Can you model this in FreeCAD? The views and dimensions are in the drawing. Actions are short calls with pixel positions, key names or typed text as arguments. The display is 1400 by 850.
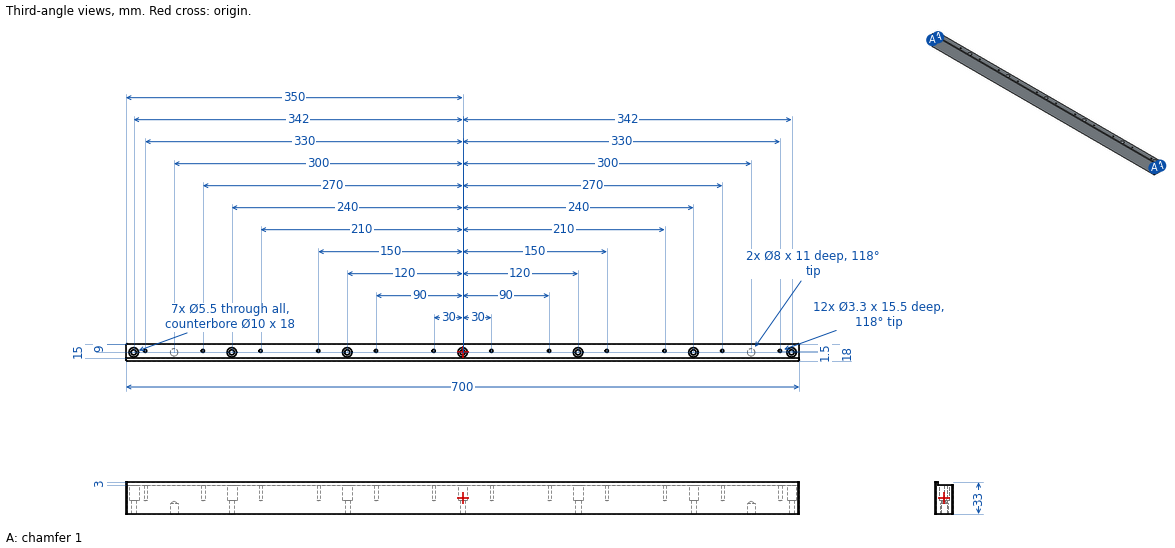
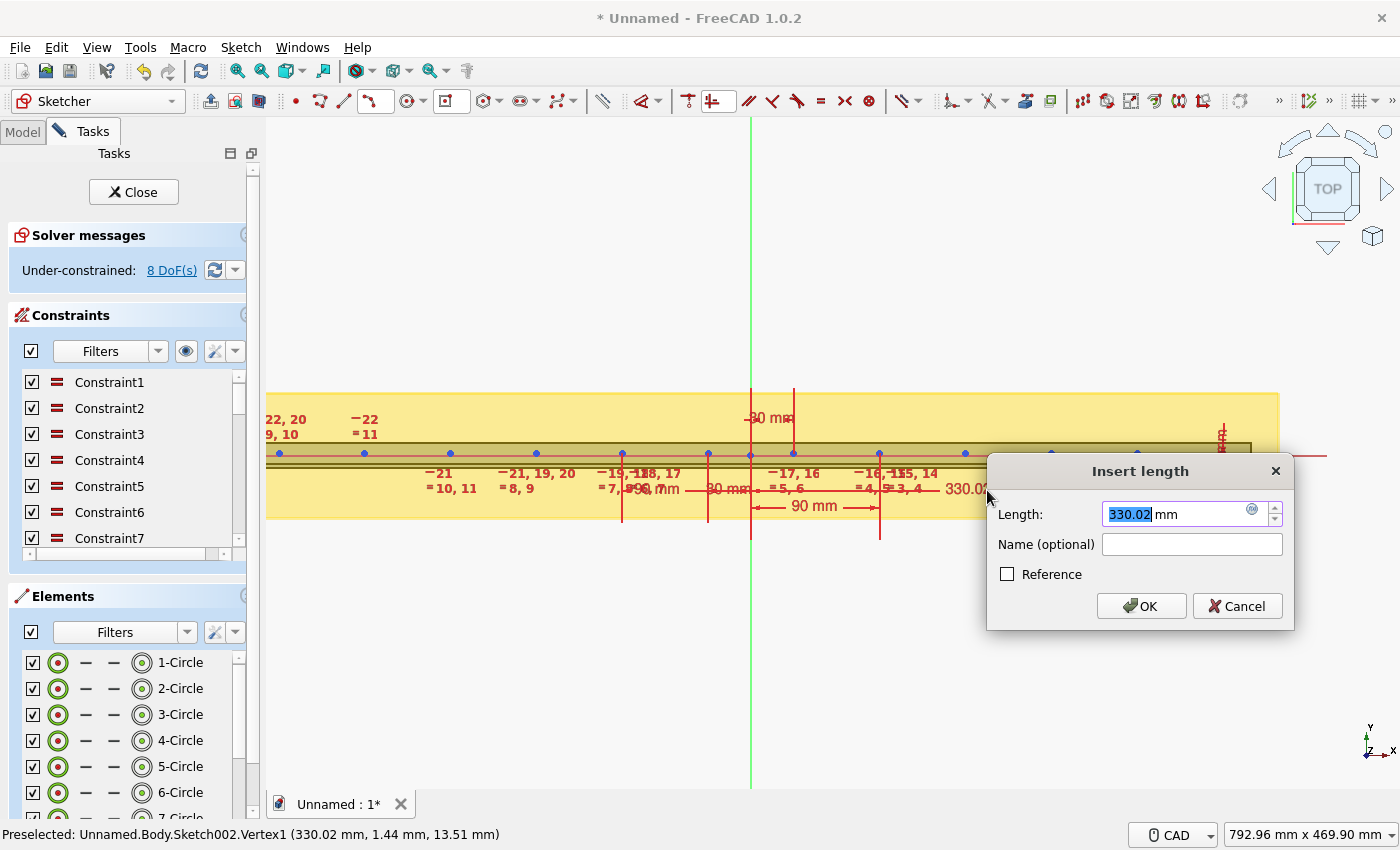
text(330)
key(Return)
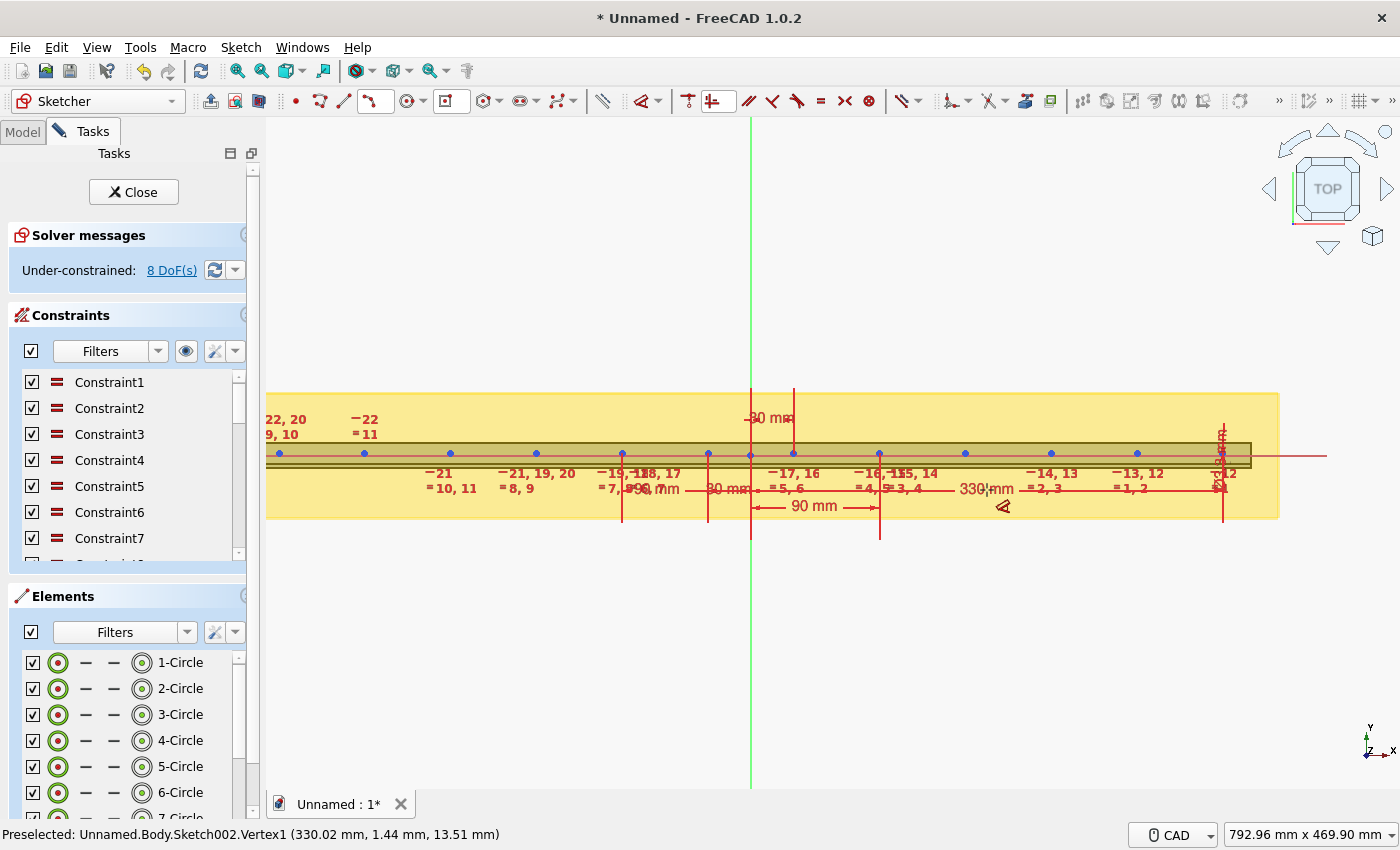
scroll(1223, 453, up, 15)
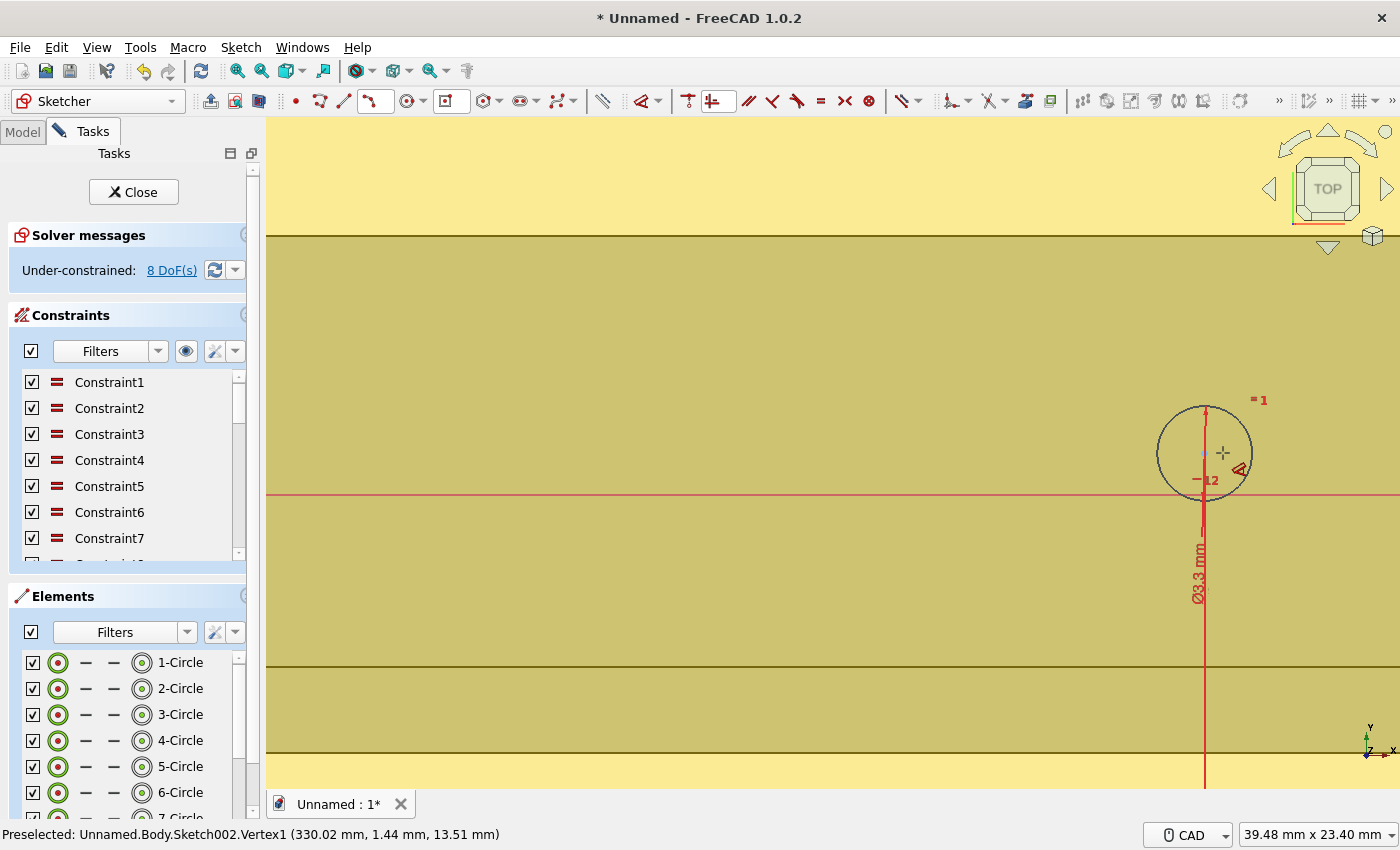
click(1205, 453)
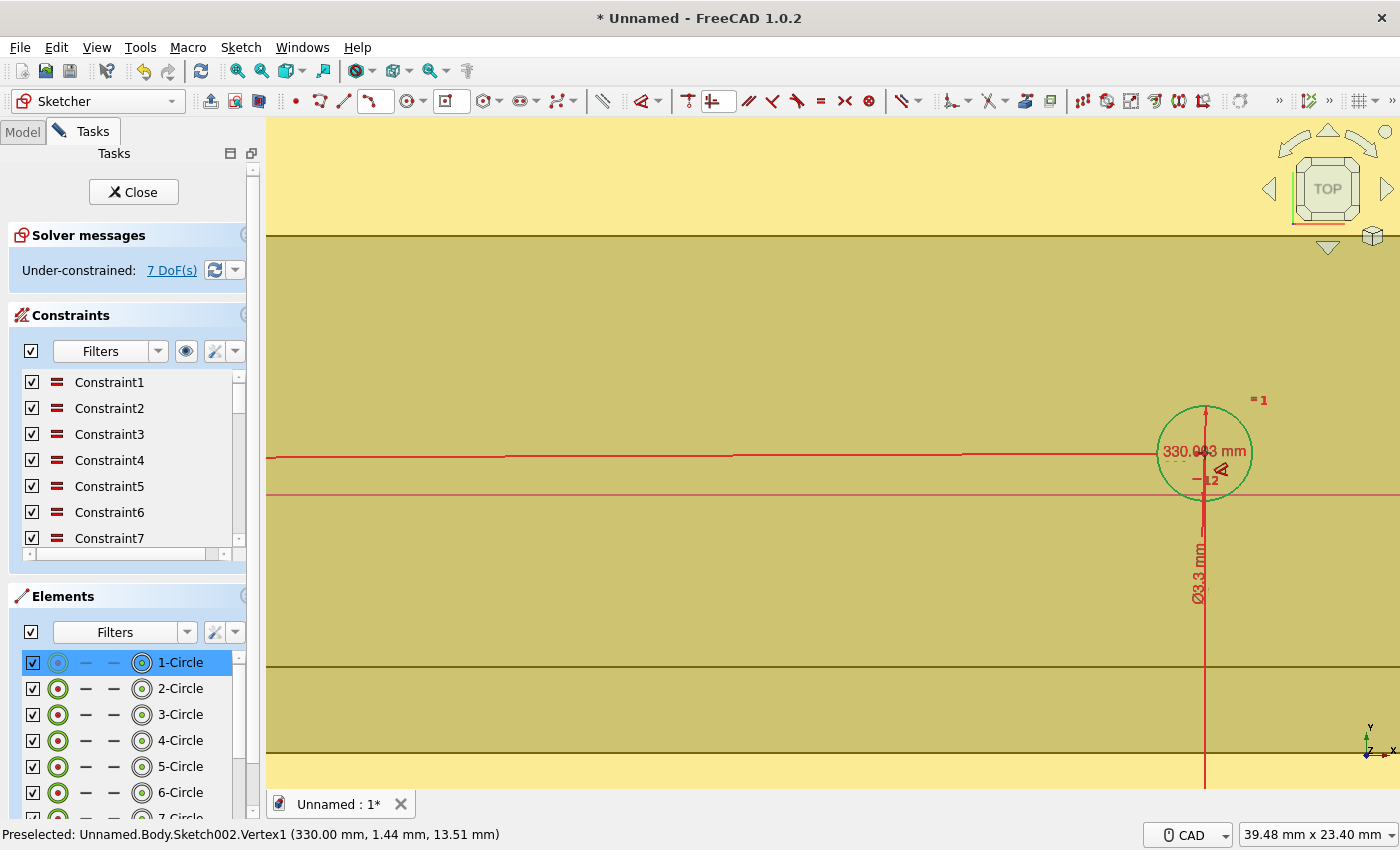
key(Escape)
key(Escape)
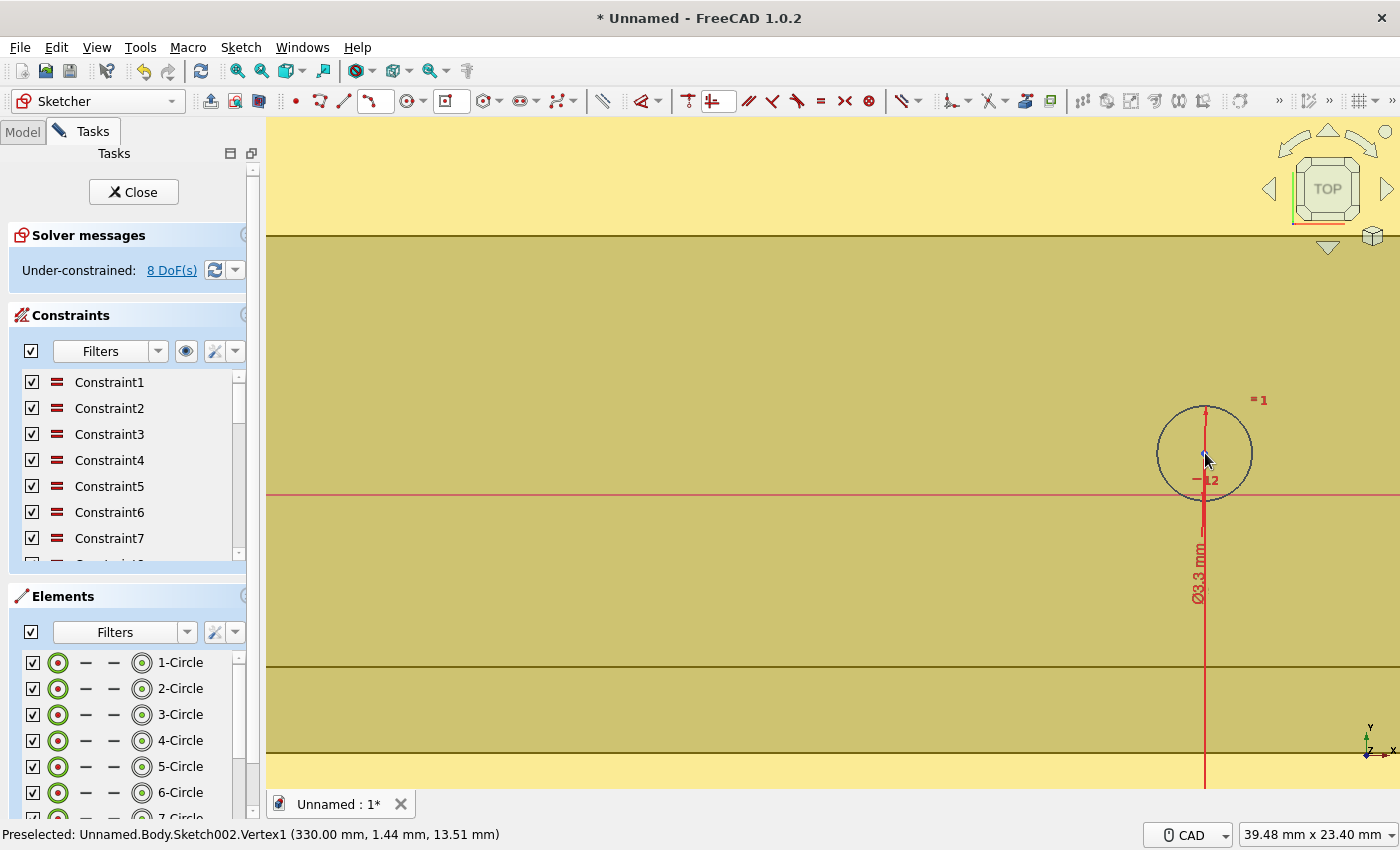
click(1205, 453)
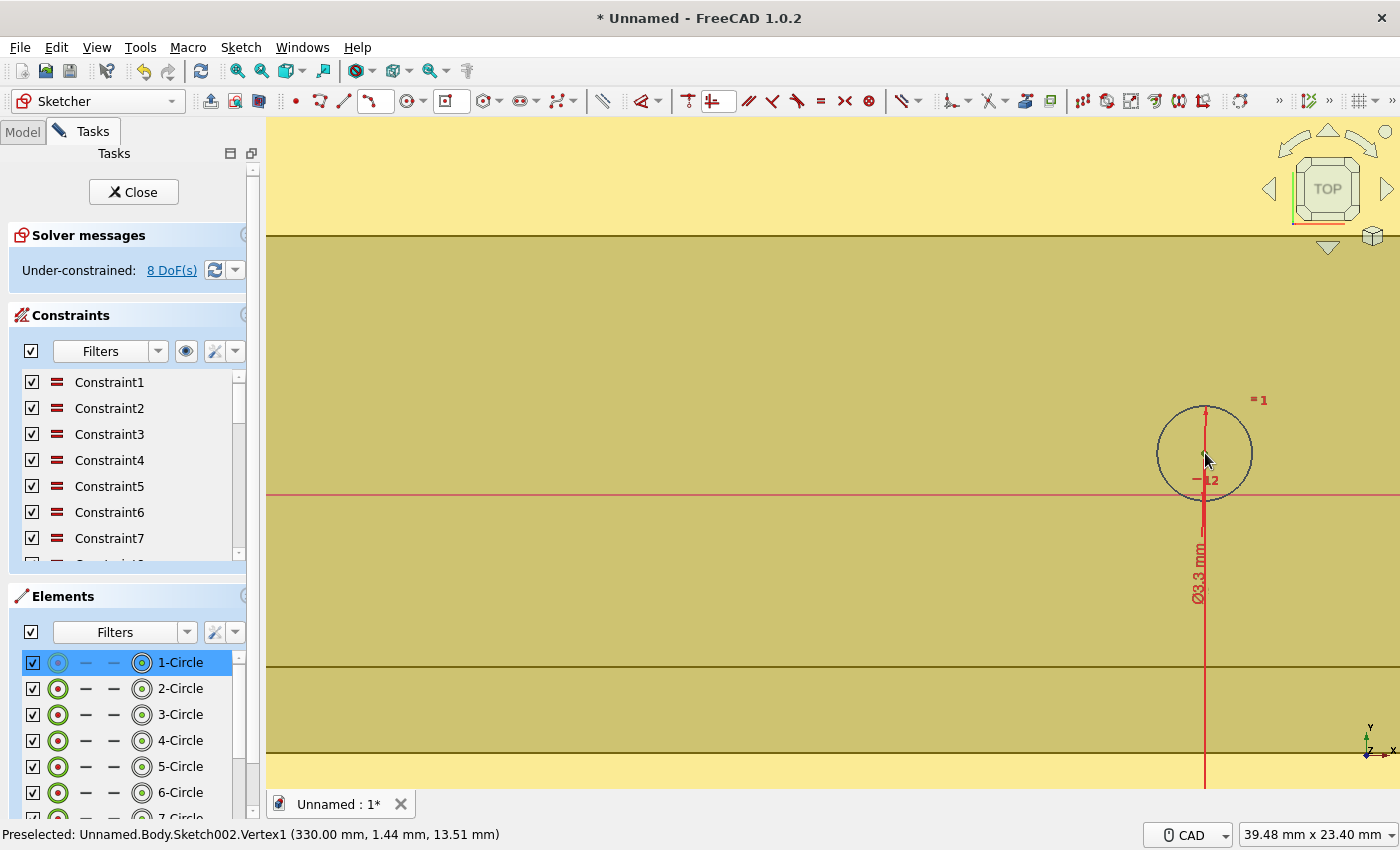
click(660, 102)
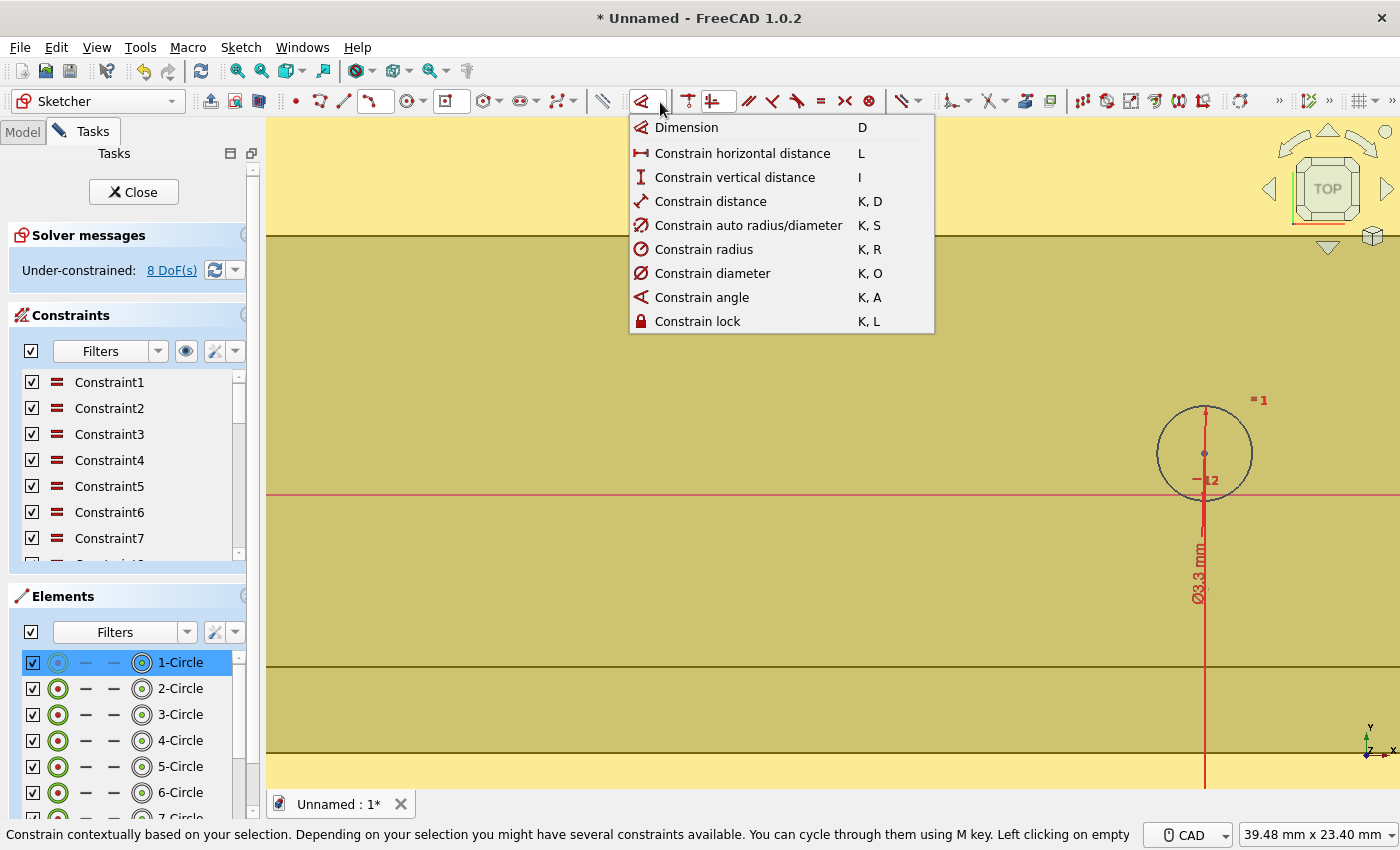
click(782, 177)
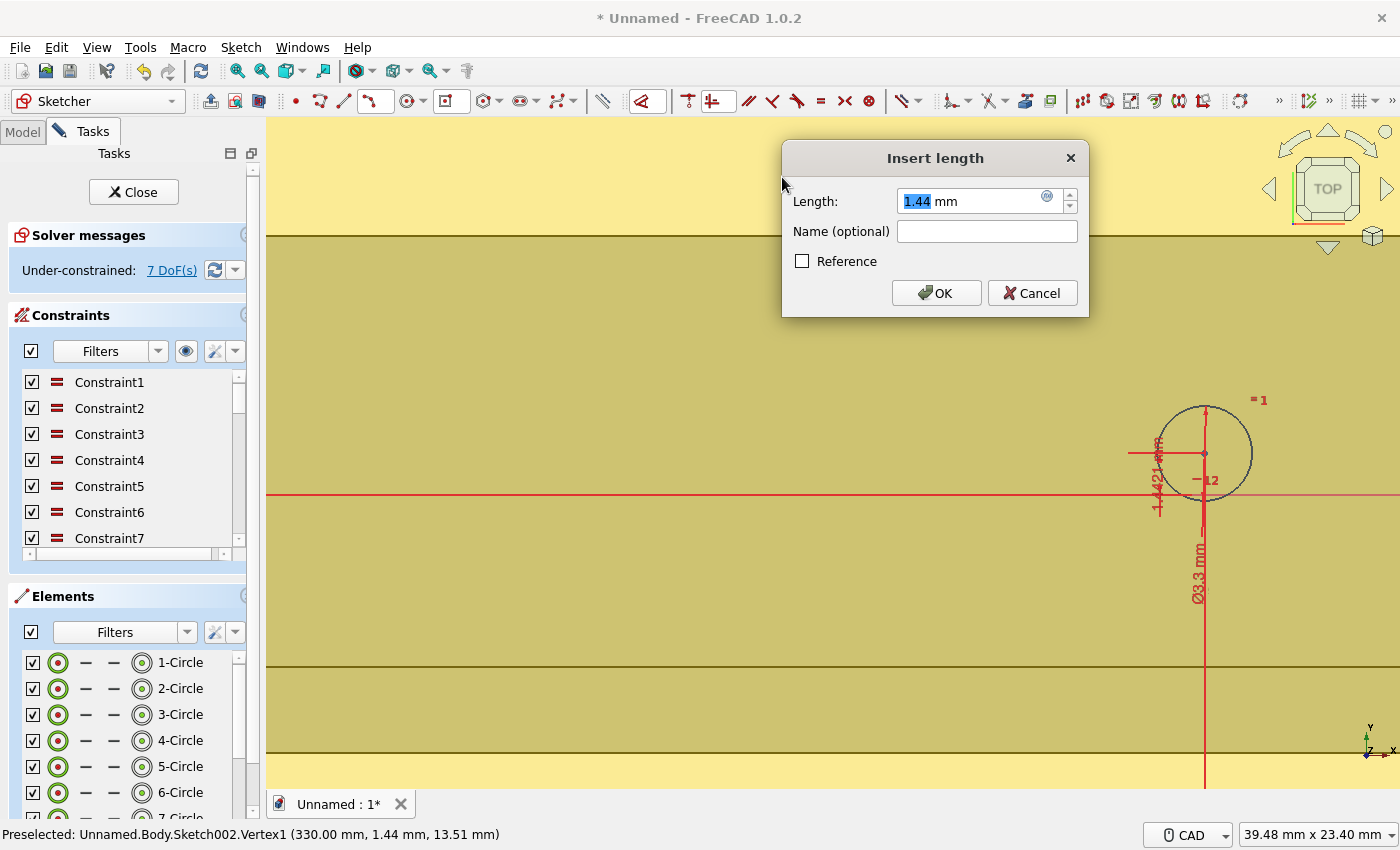
text(1.5)
key(Return)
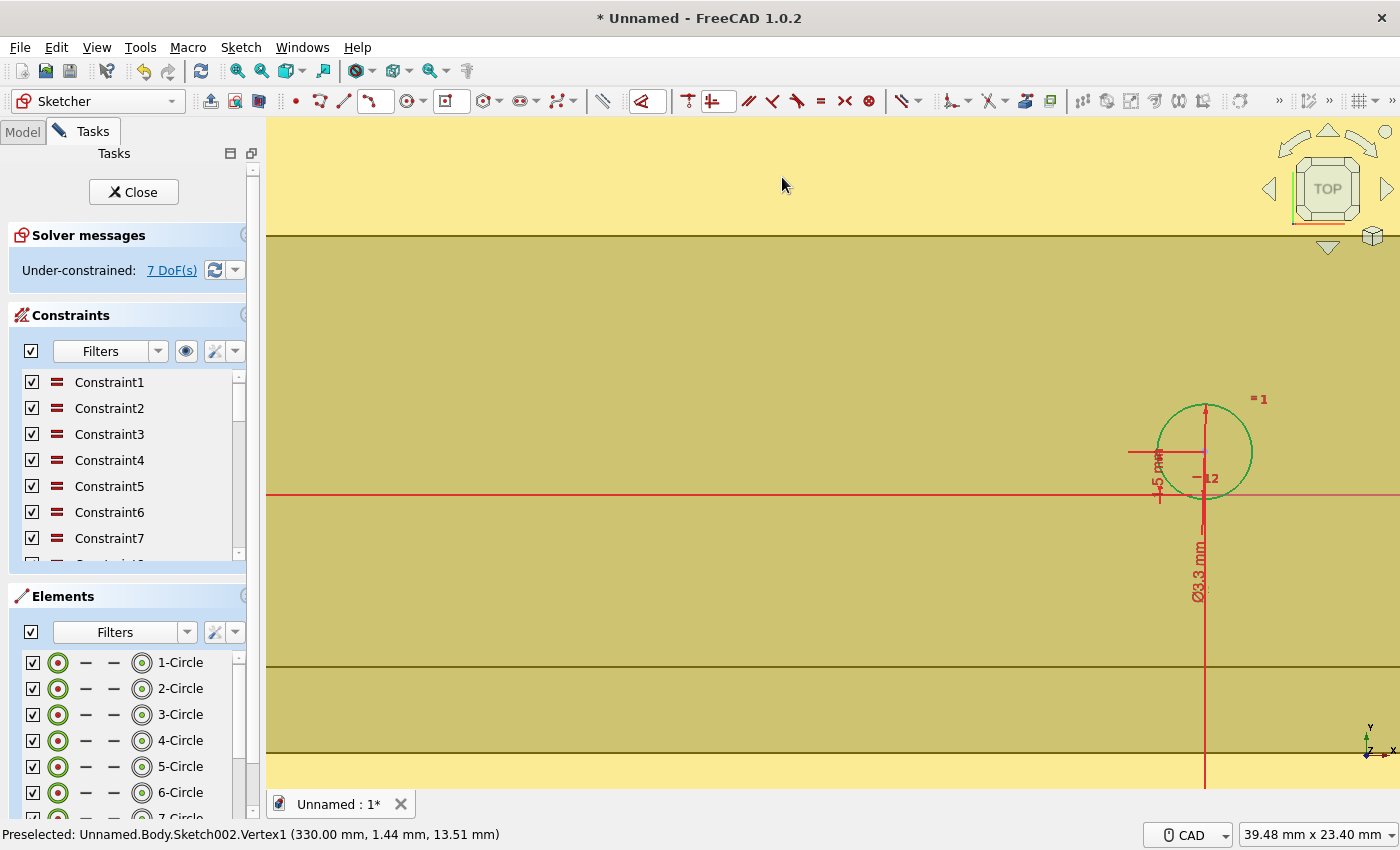
scroll(1149, 453, down, 16)